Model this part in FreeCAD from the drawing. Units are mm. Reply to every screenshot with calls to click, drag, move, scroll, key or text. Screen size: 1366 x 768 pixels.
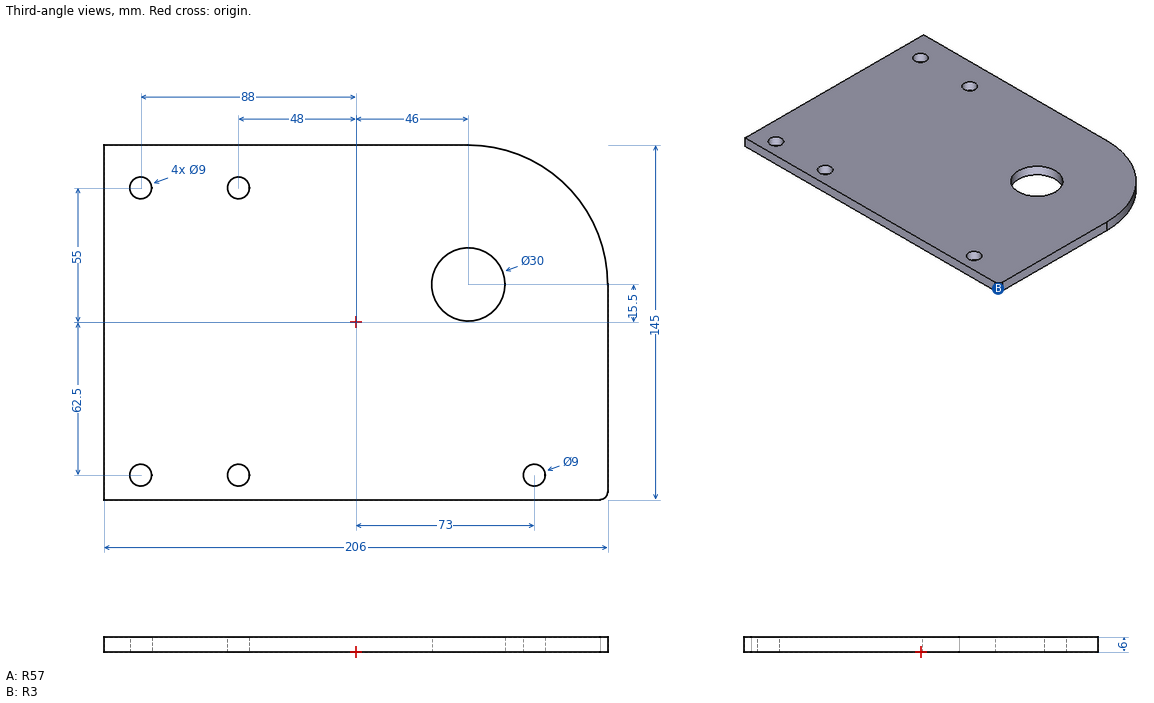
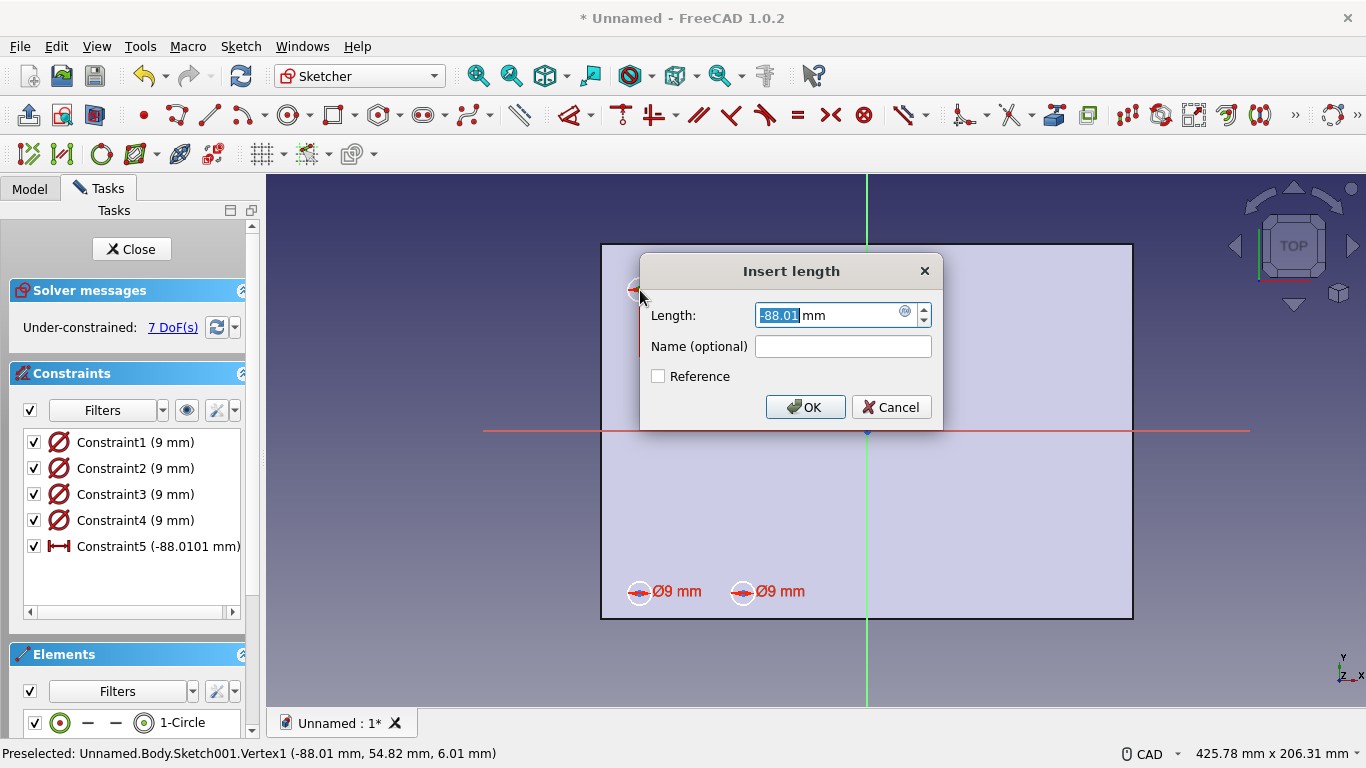
text(-88)
key(Return)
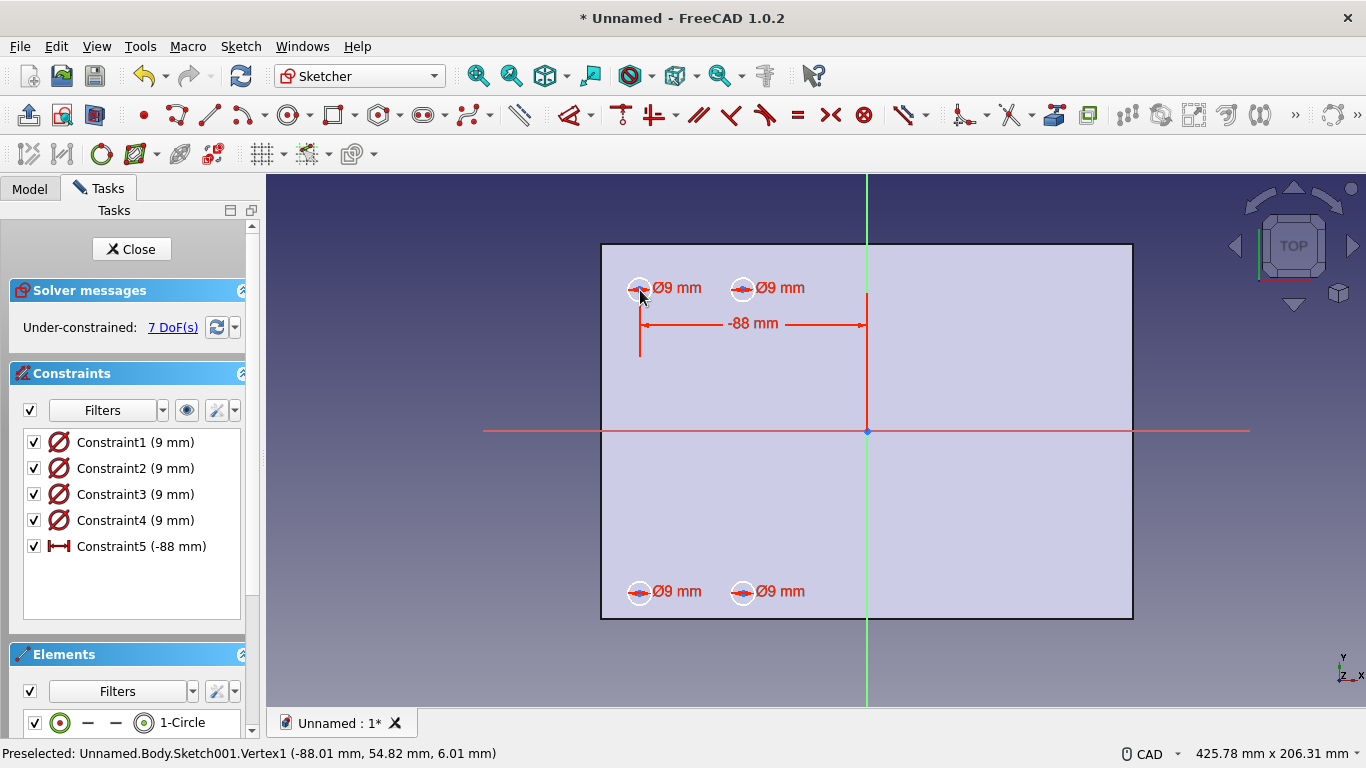
click(640, 290)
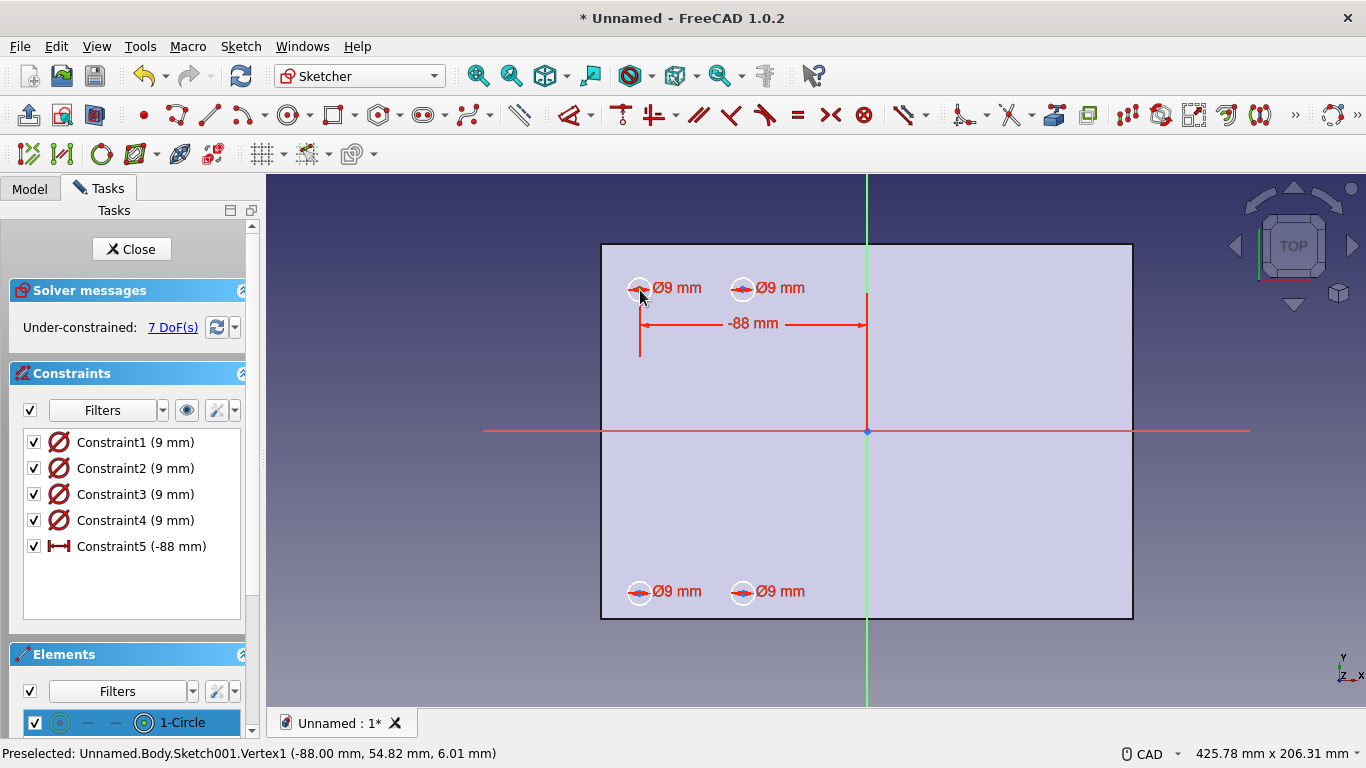
click(590, 116)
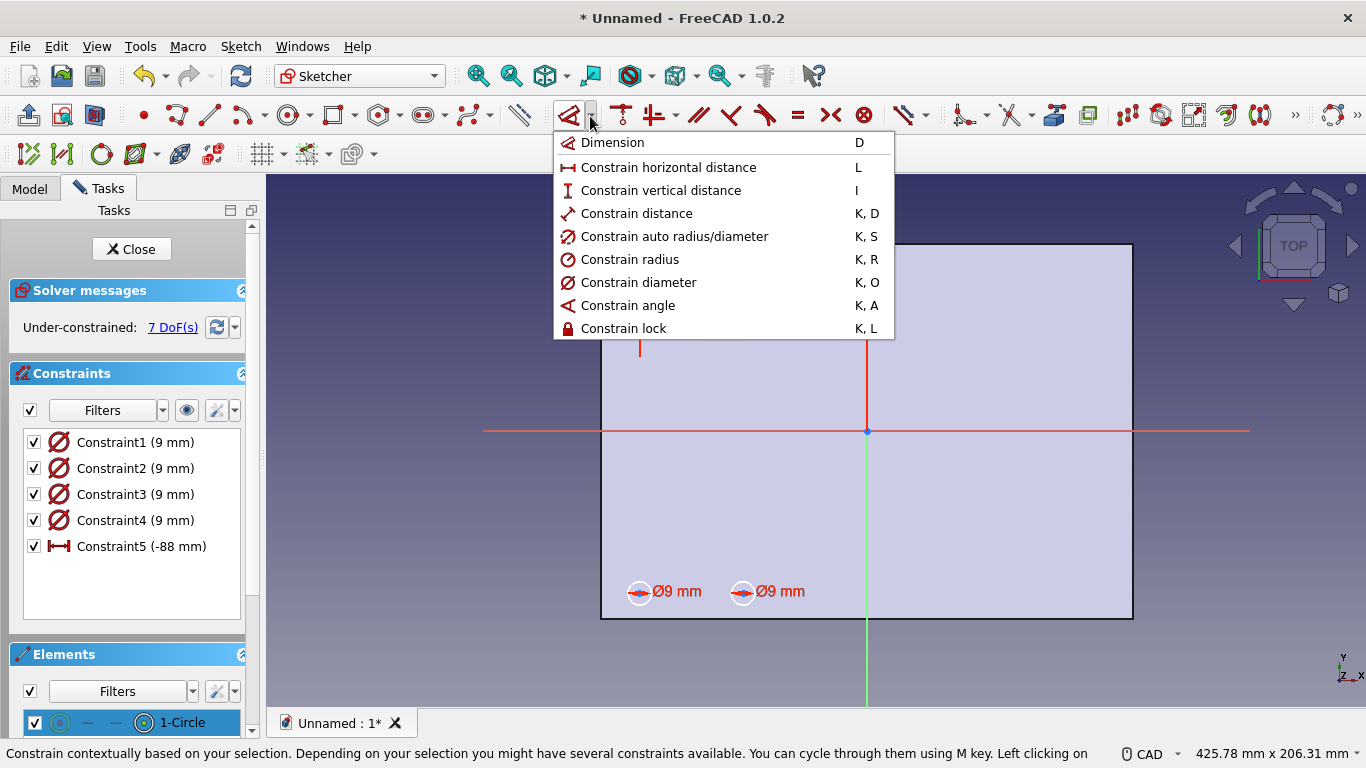
click(724, 190)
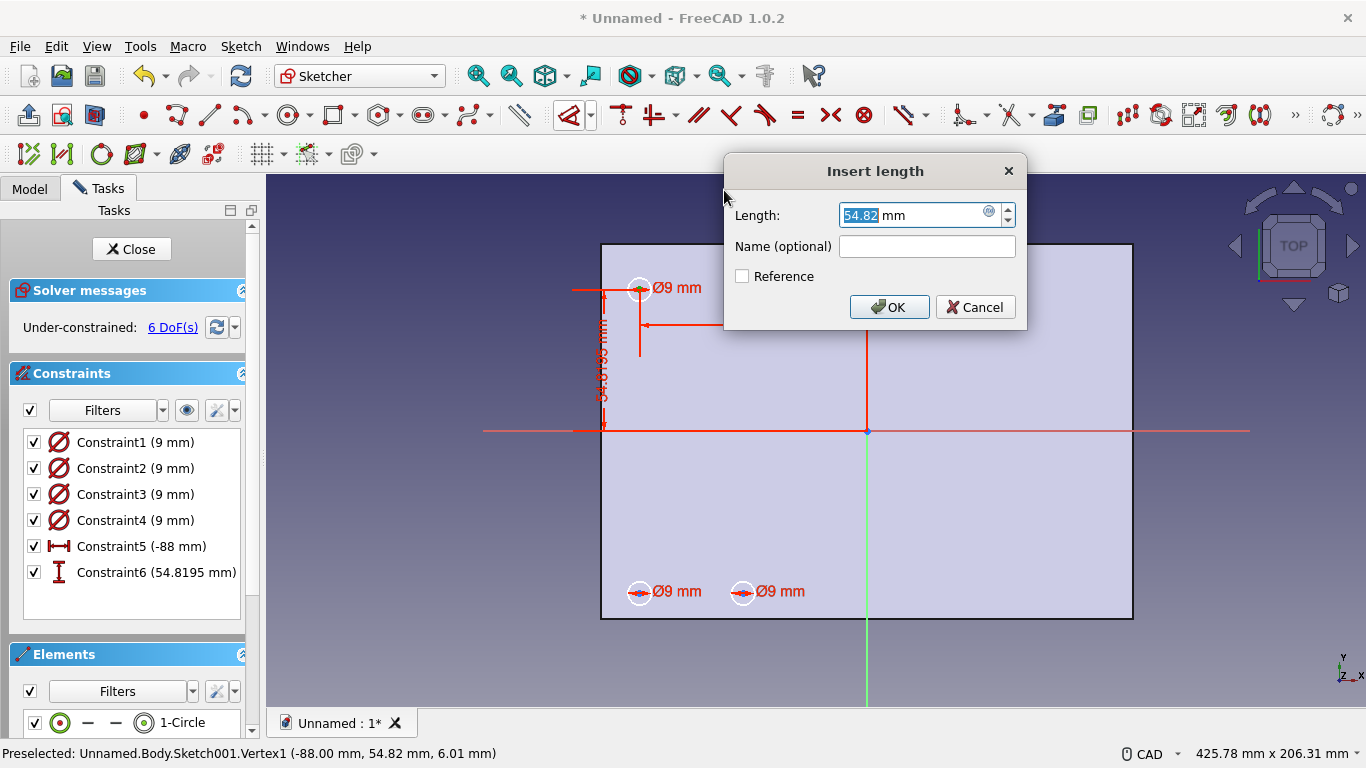
text(55)
key(Return)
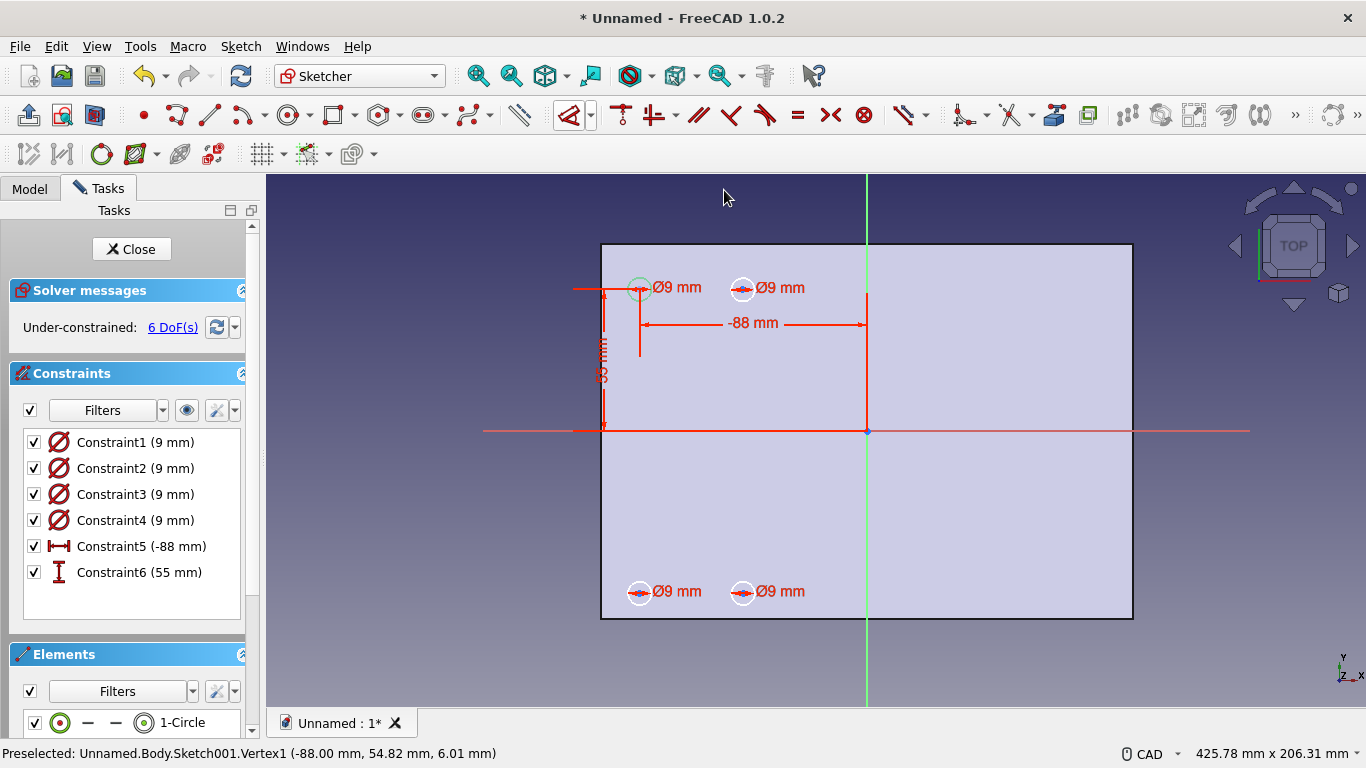
click(743, 290)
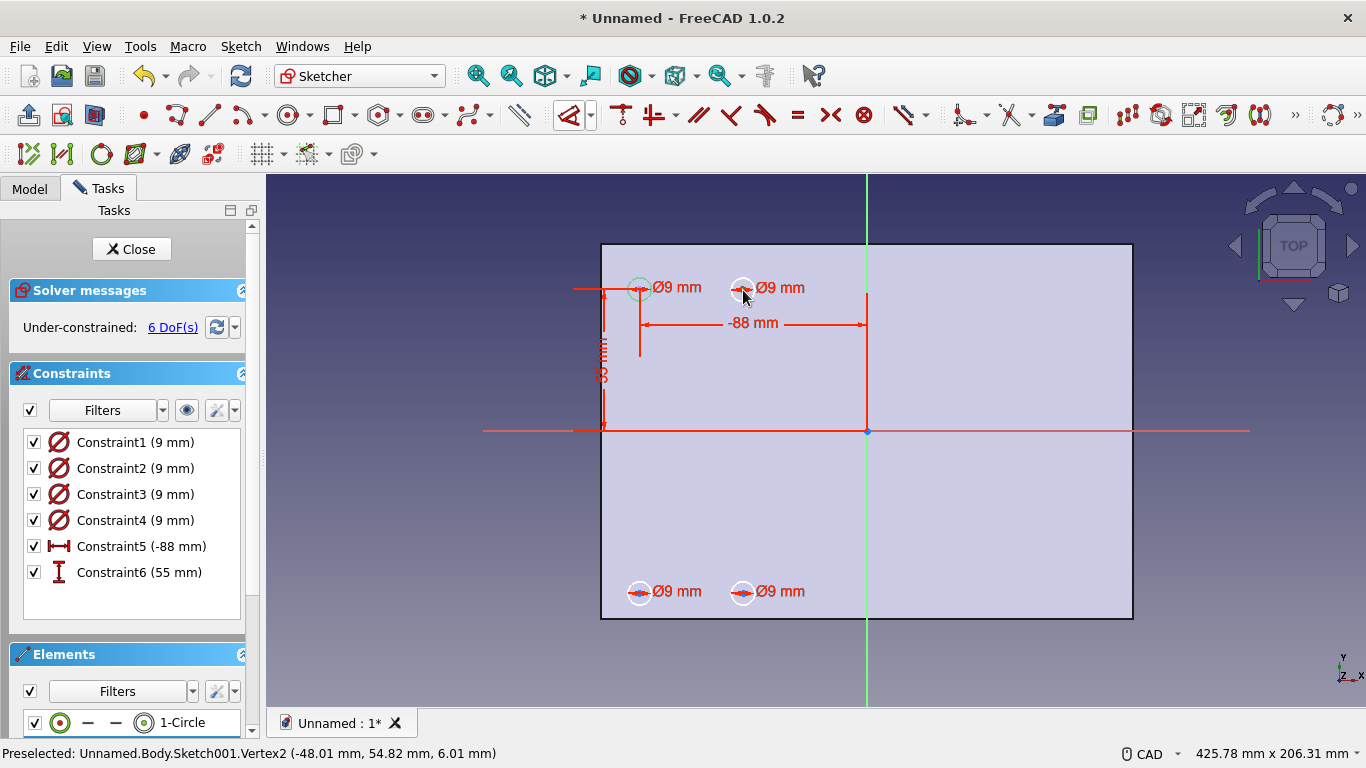
key(l)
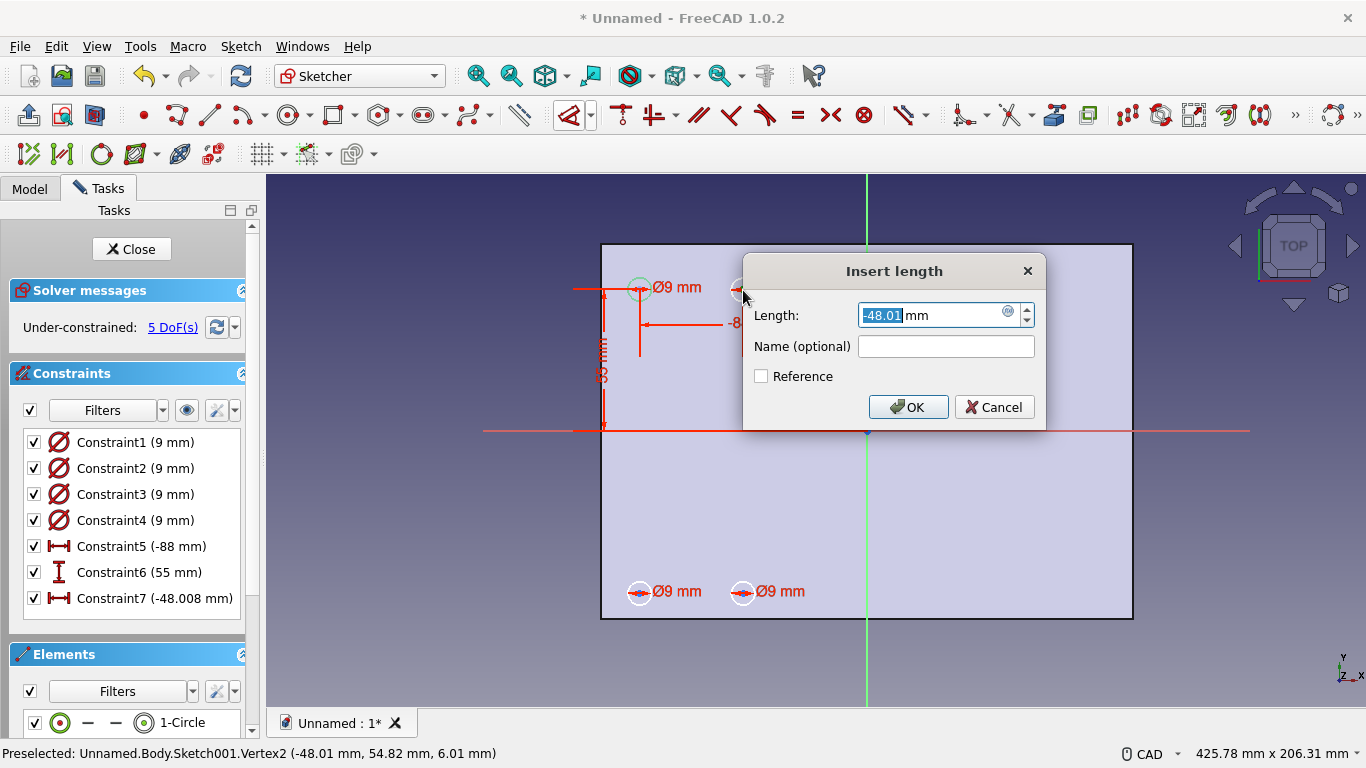
text(-48)
key(Return)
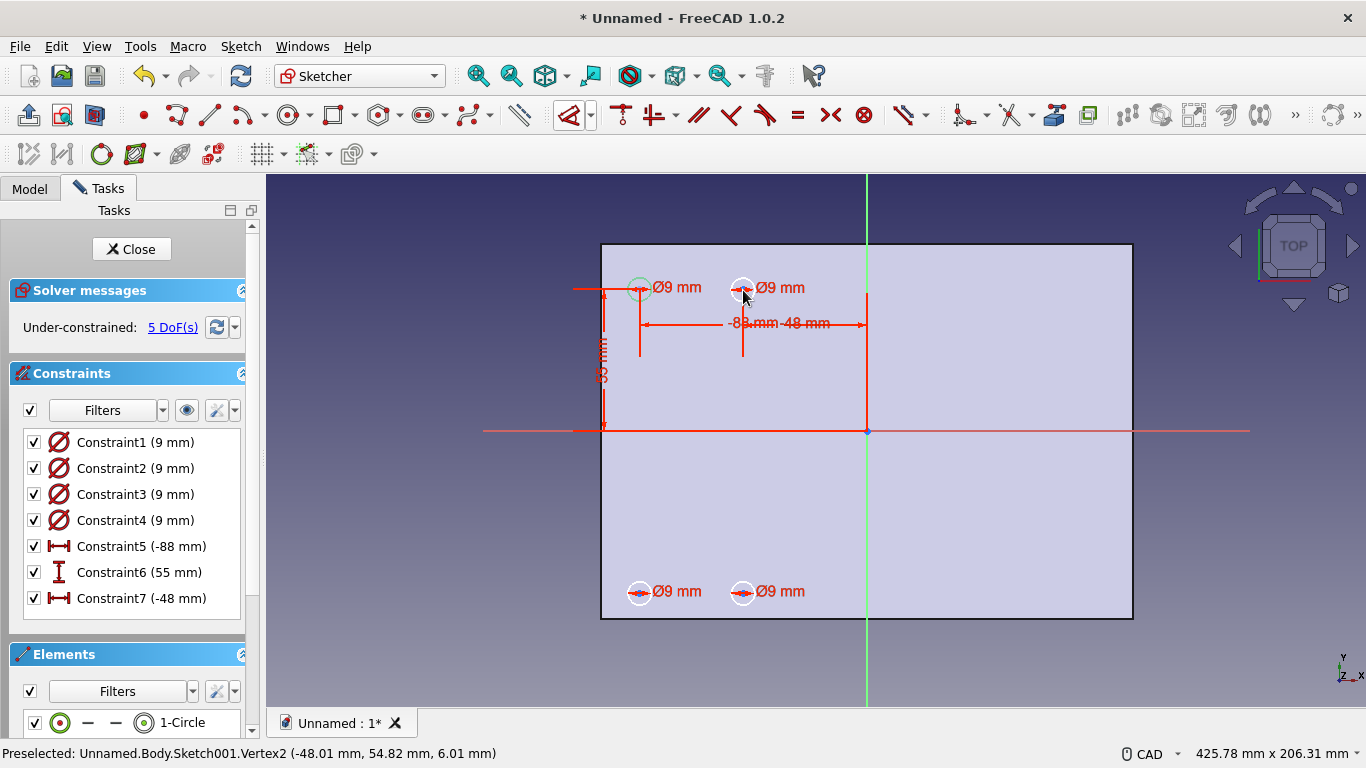
click(743, 290)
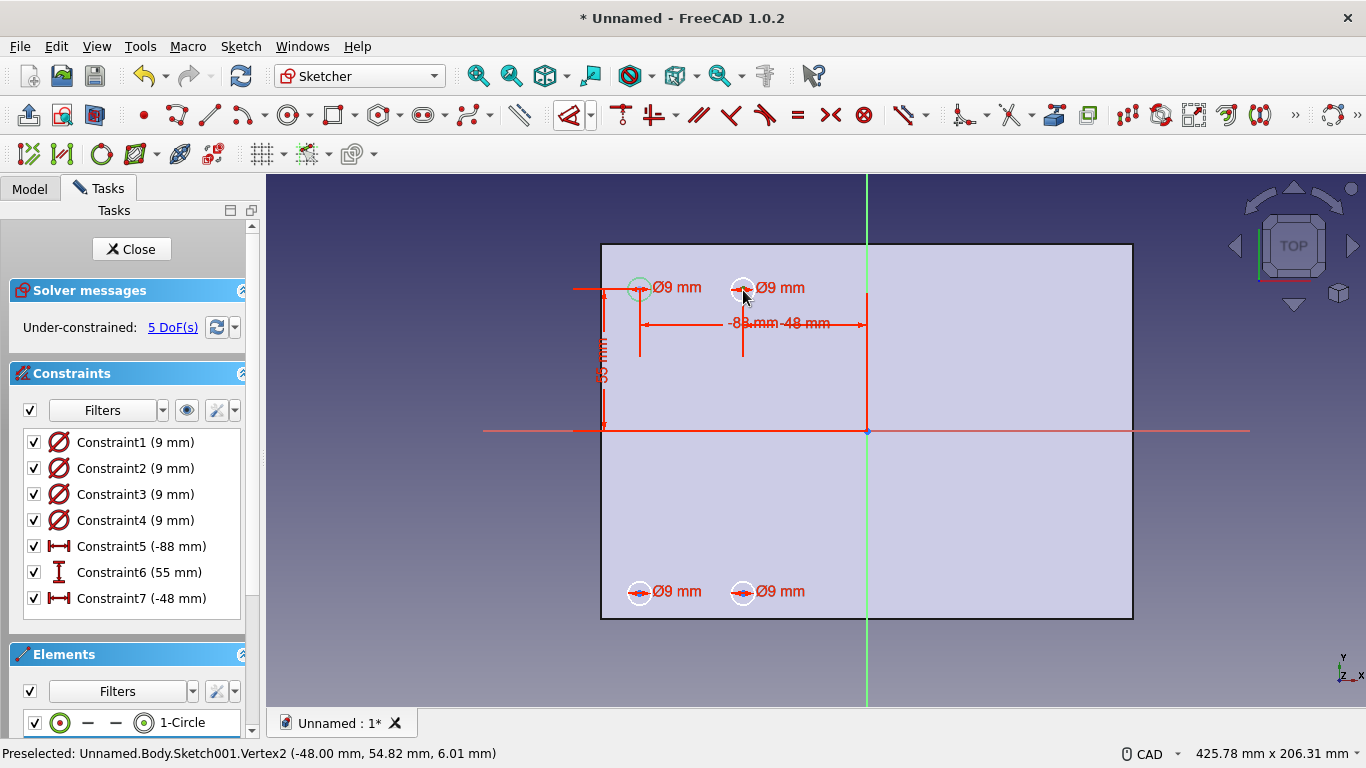
key(i)